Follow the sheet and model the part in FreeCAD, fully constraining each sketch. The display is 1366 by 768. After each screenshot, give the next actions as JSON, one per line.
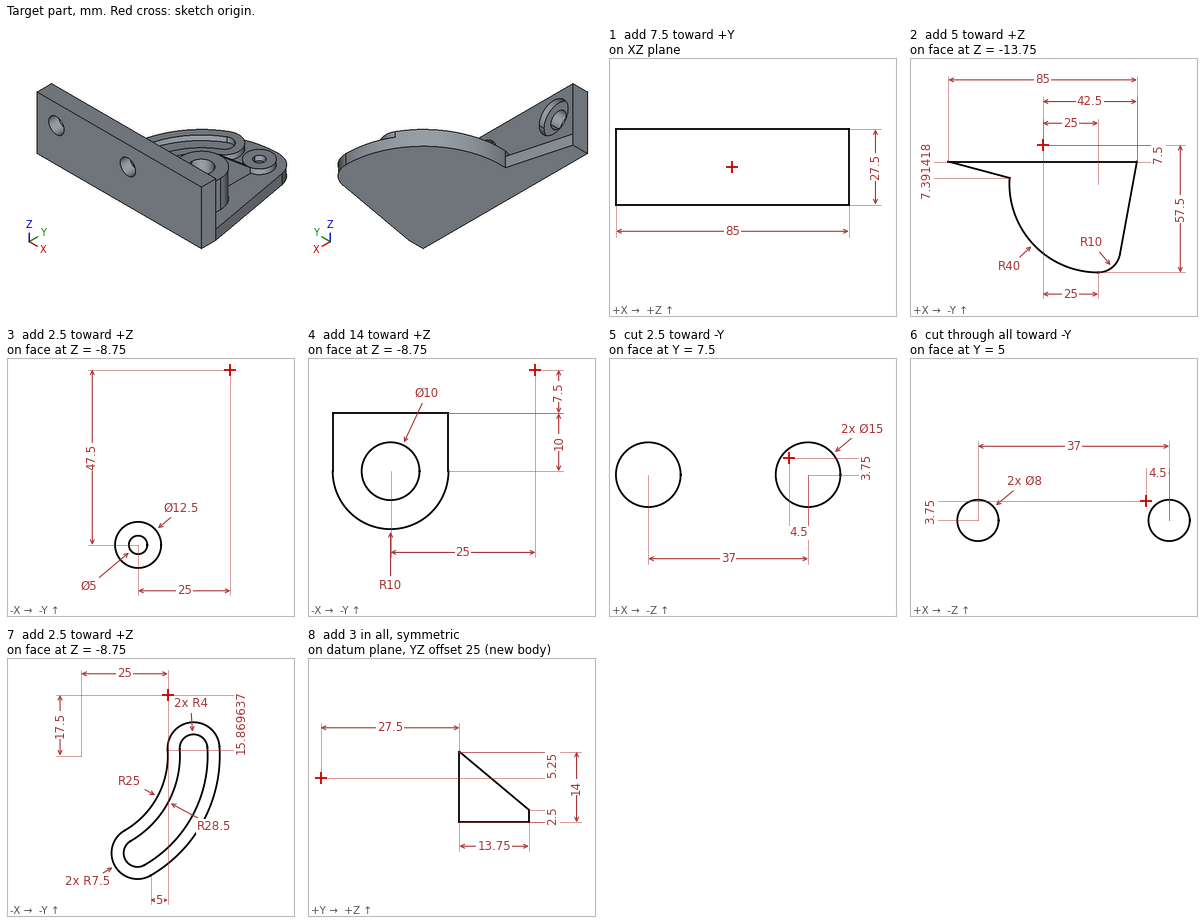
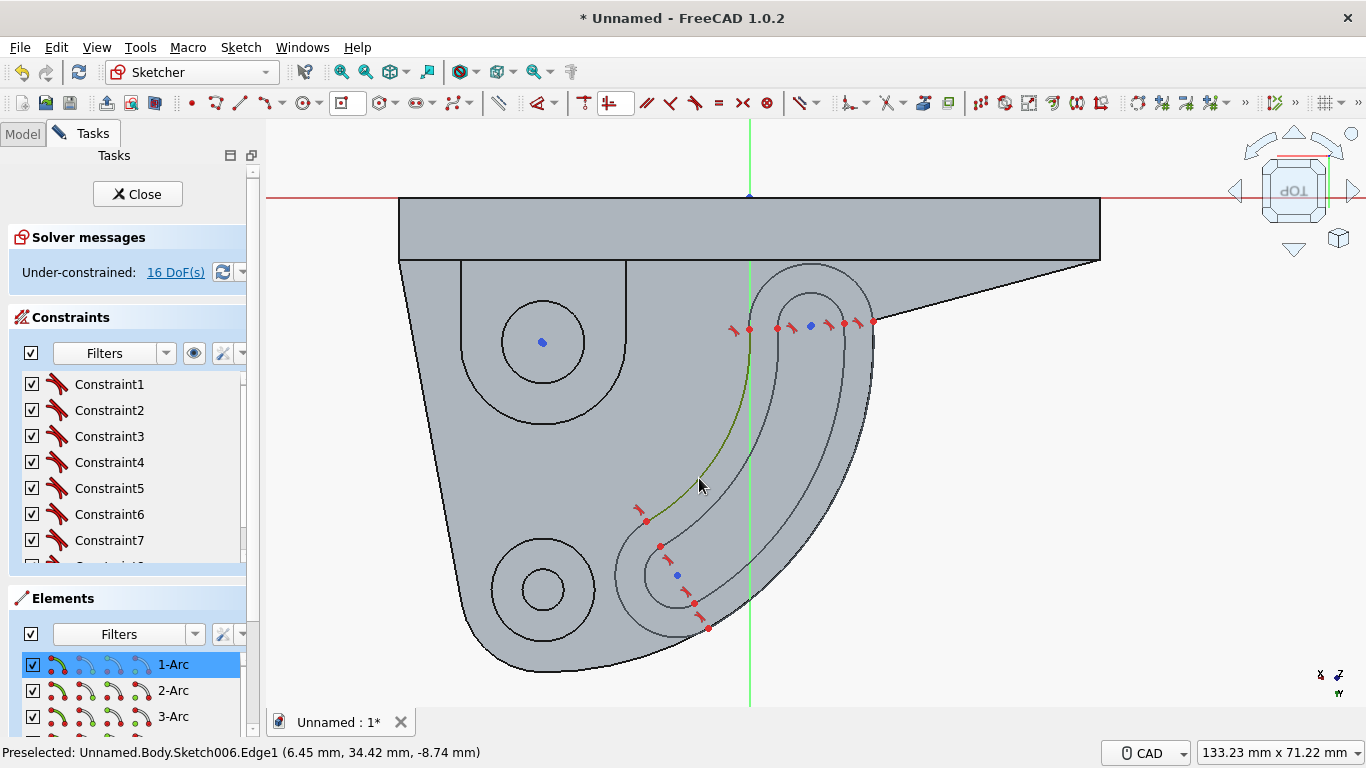
{"action": "left_click", "coordinate": [792, 559]}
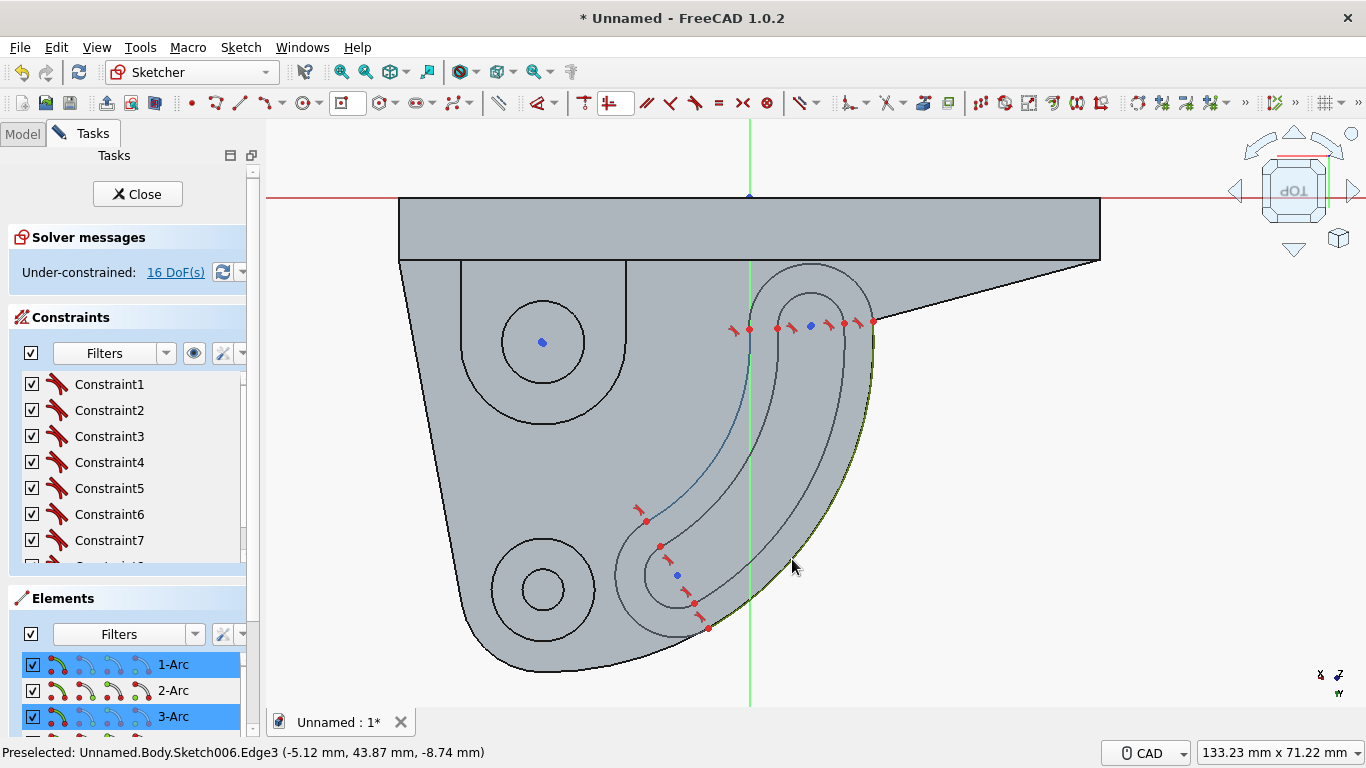
{"action": "left_click", "coordinate": [584, 104]}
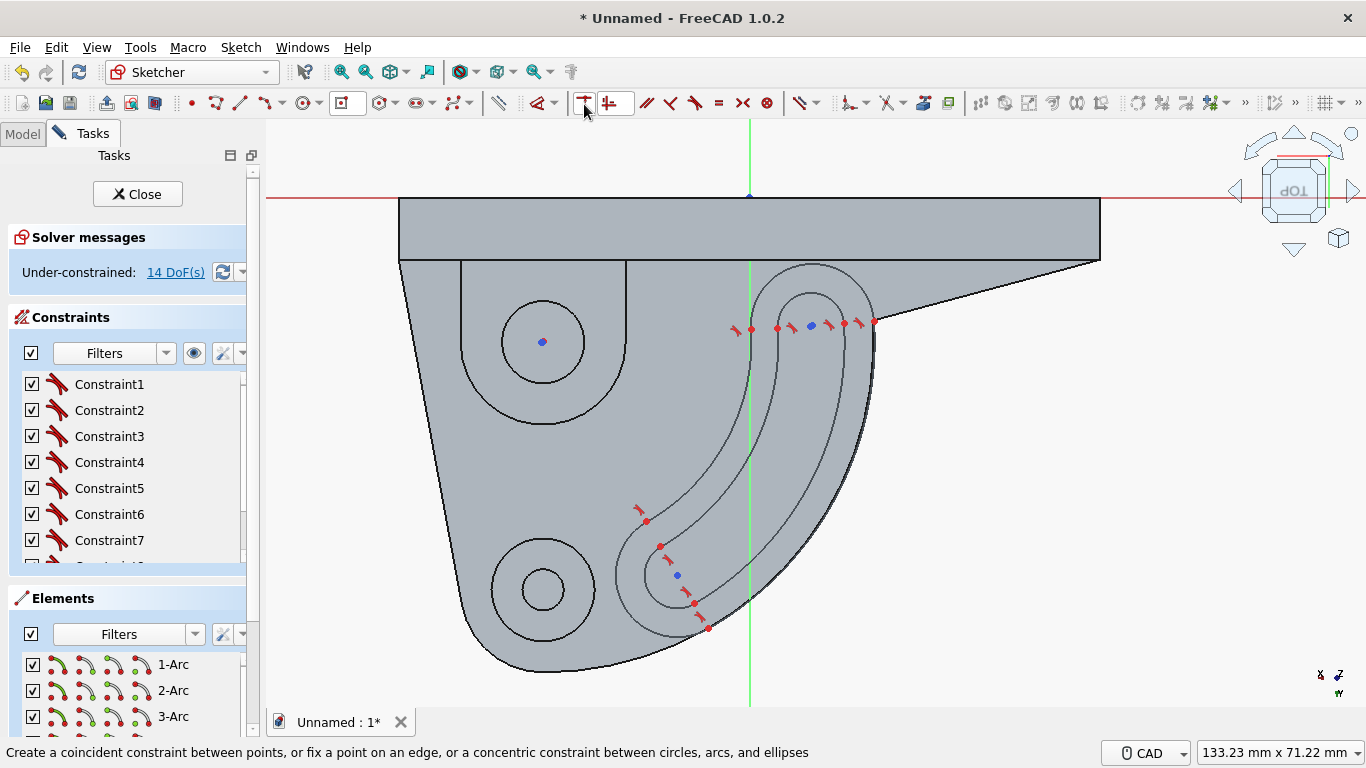
{"action": "left_click", "coordinate": [846, 274]}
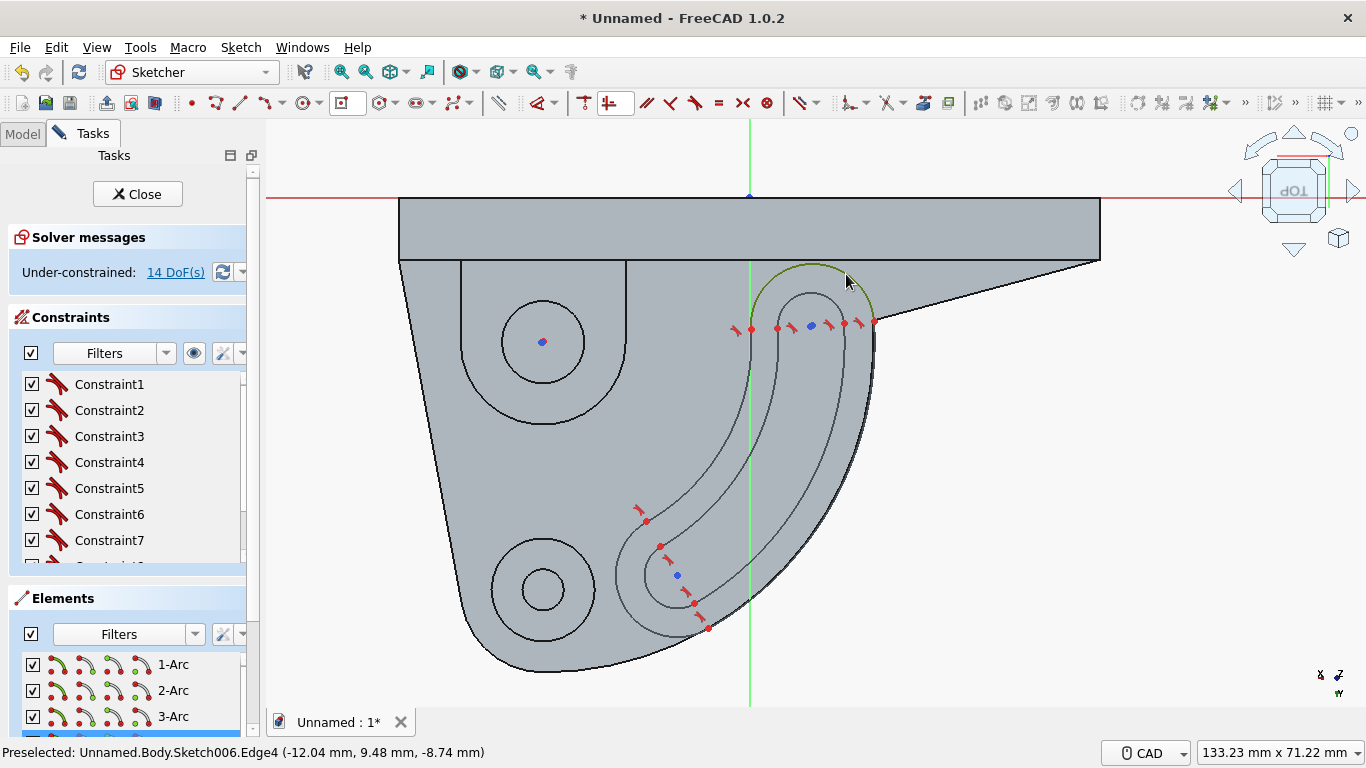
{"action": "left_click", "coordinate": [829, 298]}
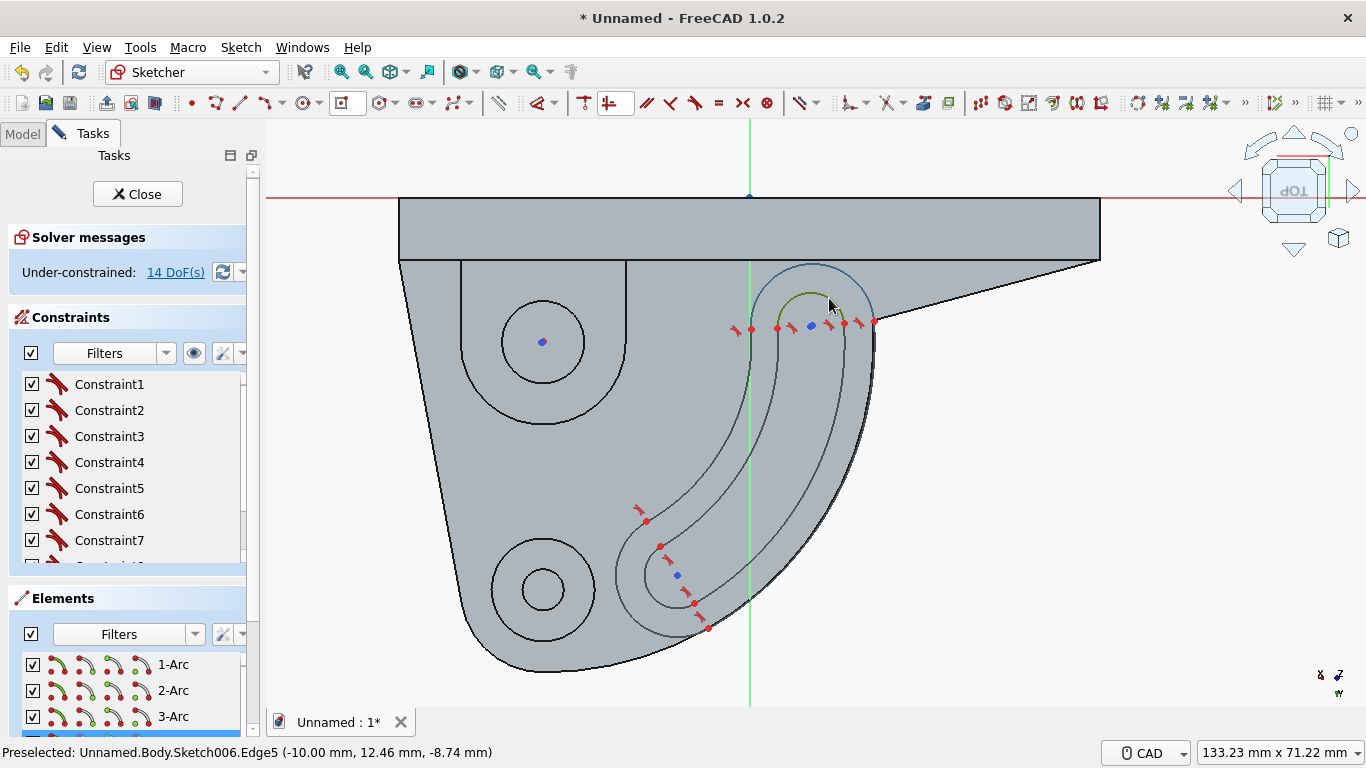
{"action": "left_click", "coordinate": [584, 104]}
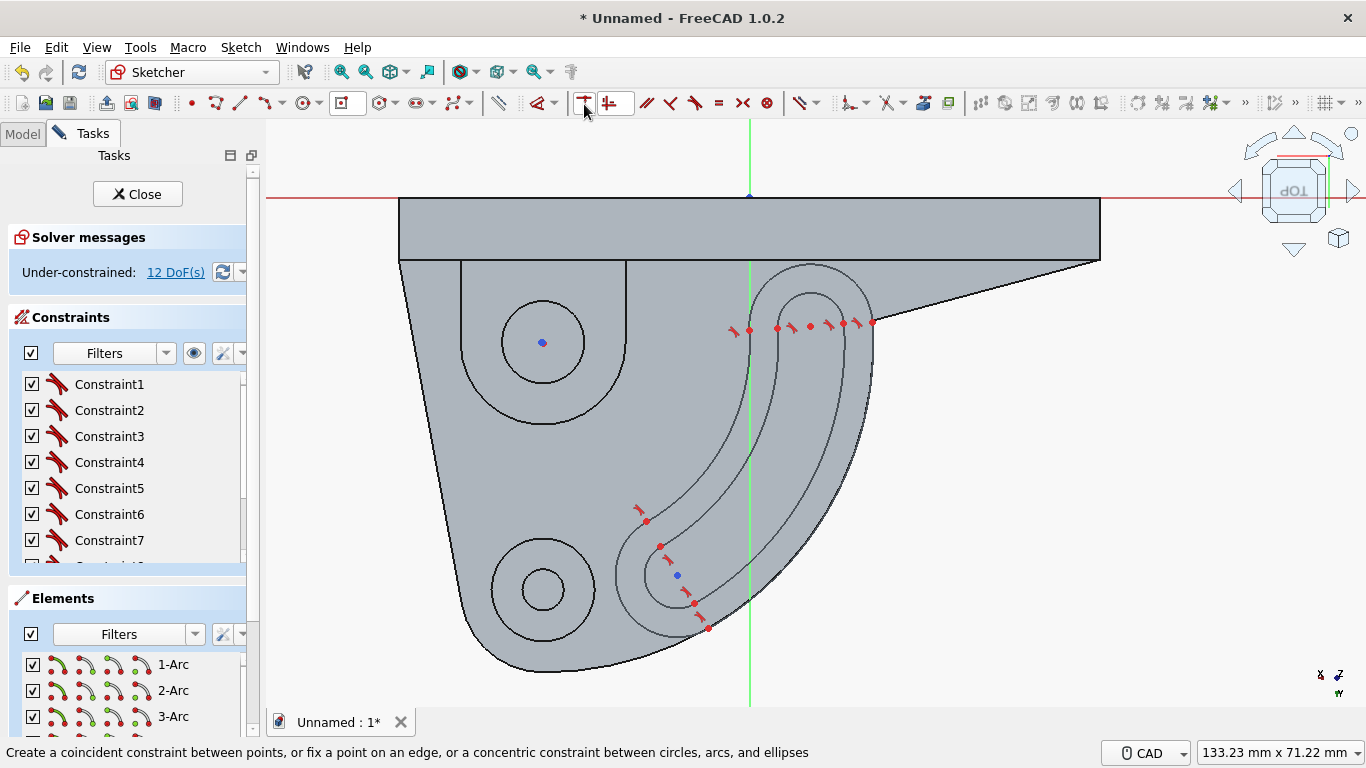
{"action": "left_click", "coordinate": [699, 478]}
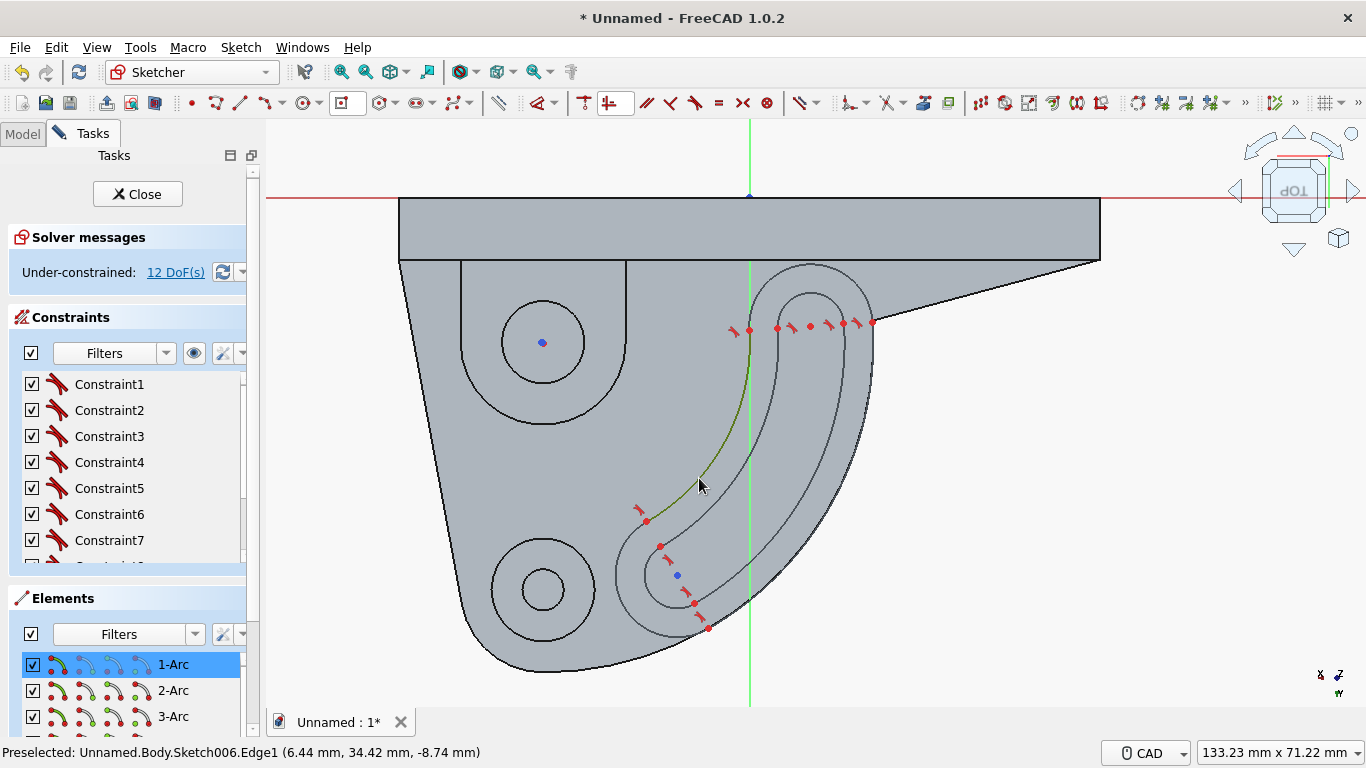
{"action": "left_click", "coordinate": [771, 540]}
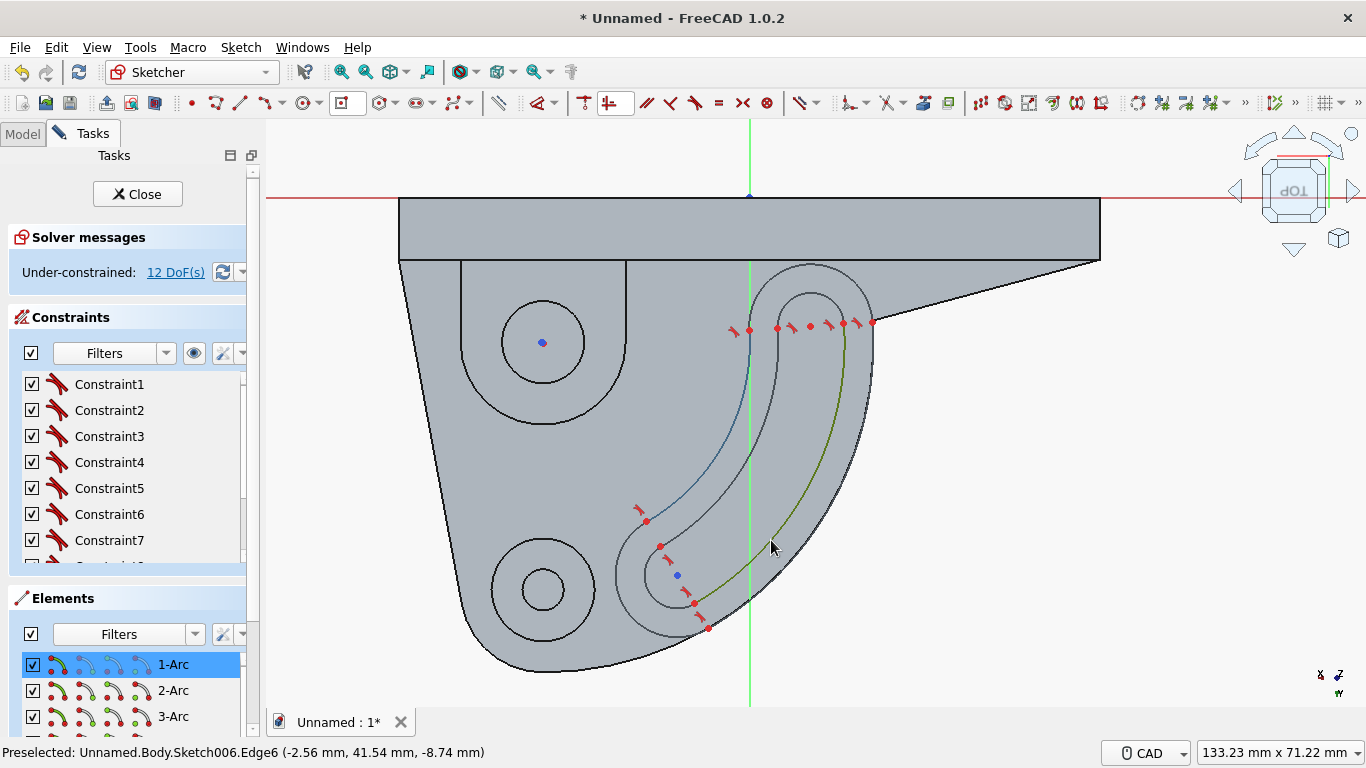
{"action": "left_click", "coordinate": [584, 104]}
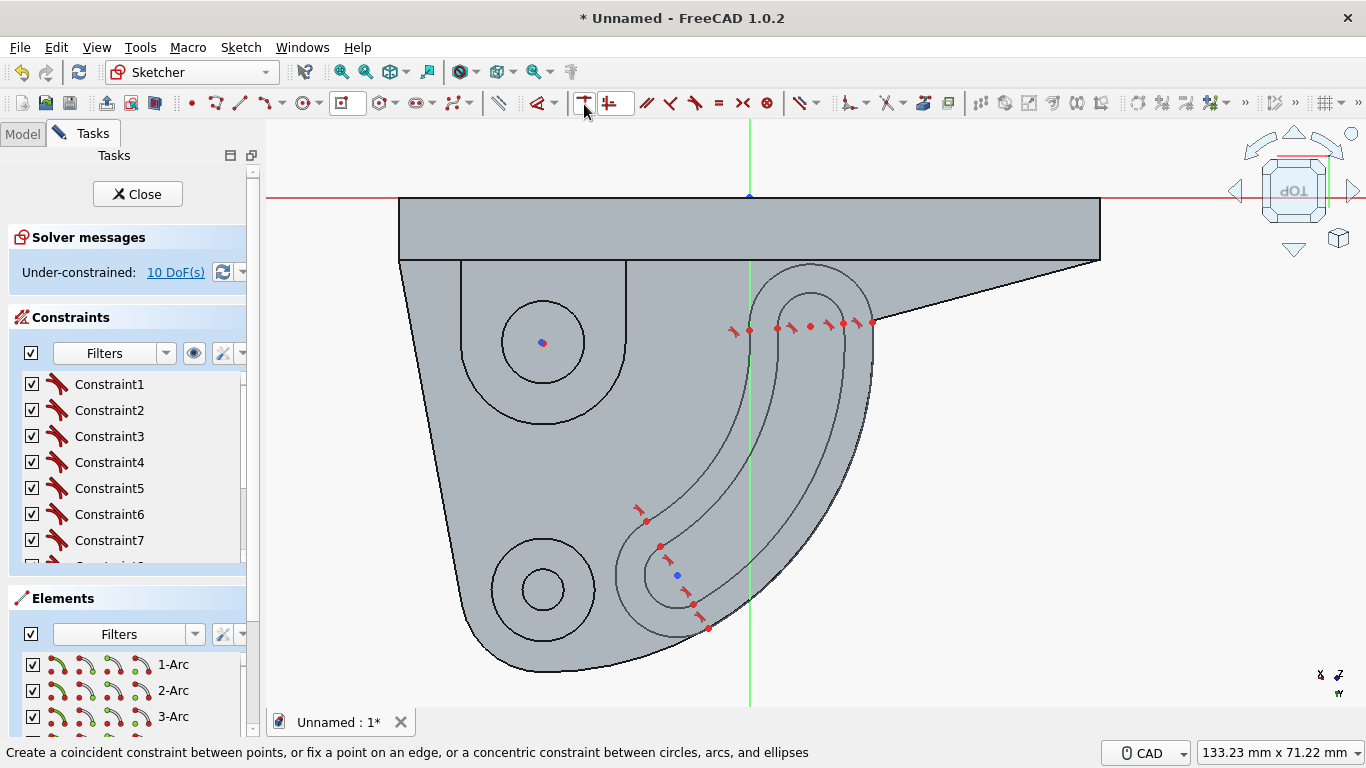
{"action": "left_click", "coordinate": [616, 569]}